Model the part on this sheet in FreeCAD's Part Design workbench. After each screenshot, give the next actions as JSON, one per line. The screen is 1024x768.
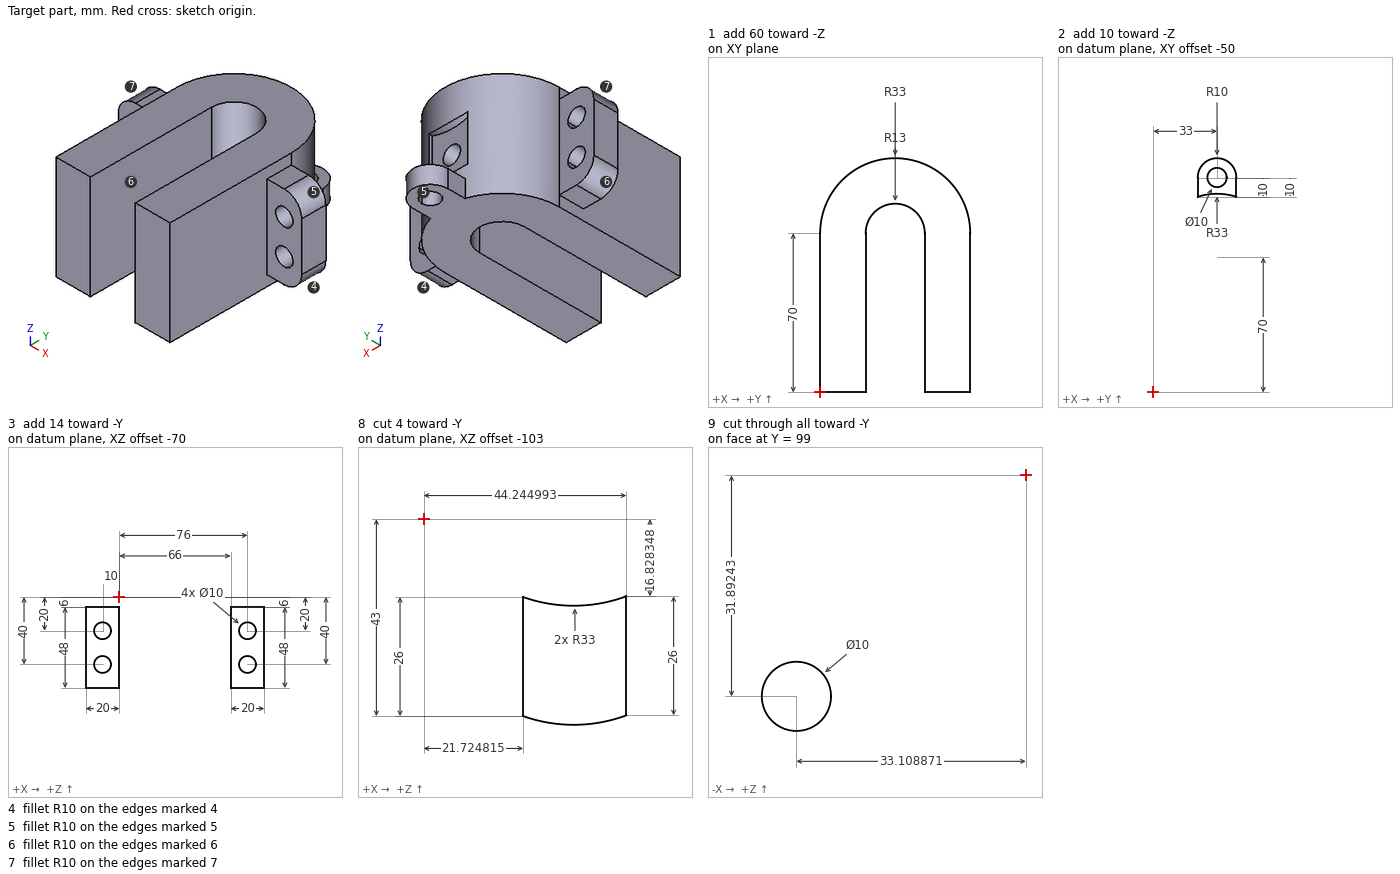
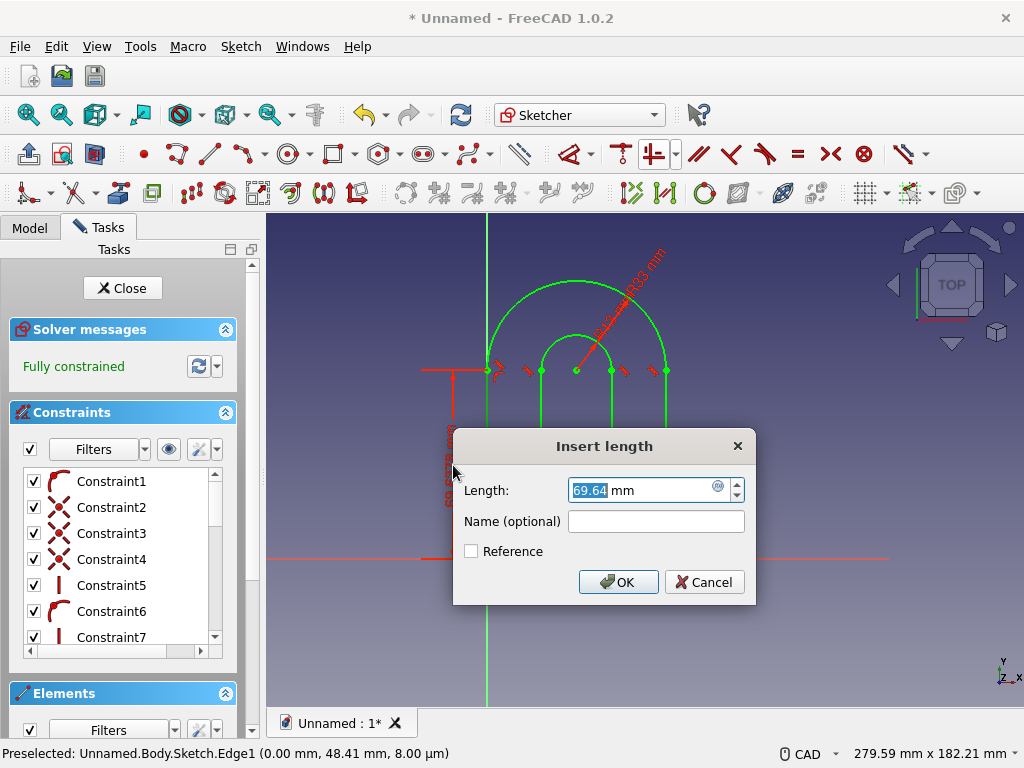
{"action": "type", "text": "70"}
{"action": "key", "text": "Return"}
{"action": "key", "text": "Escape"}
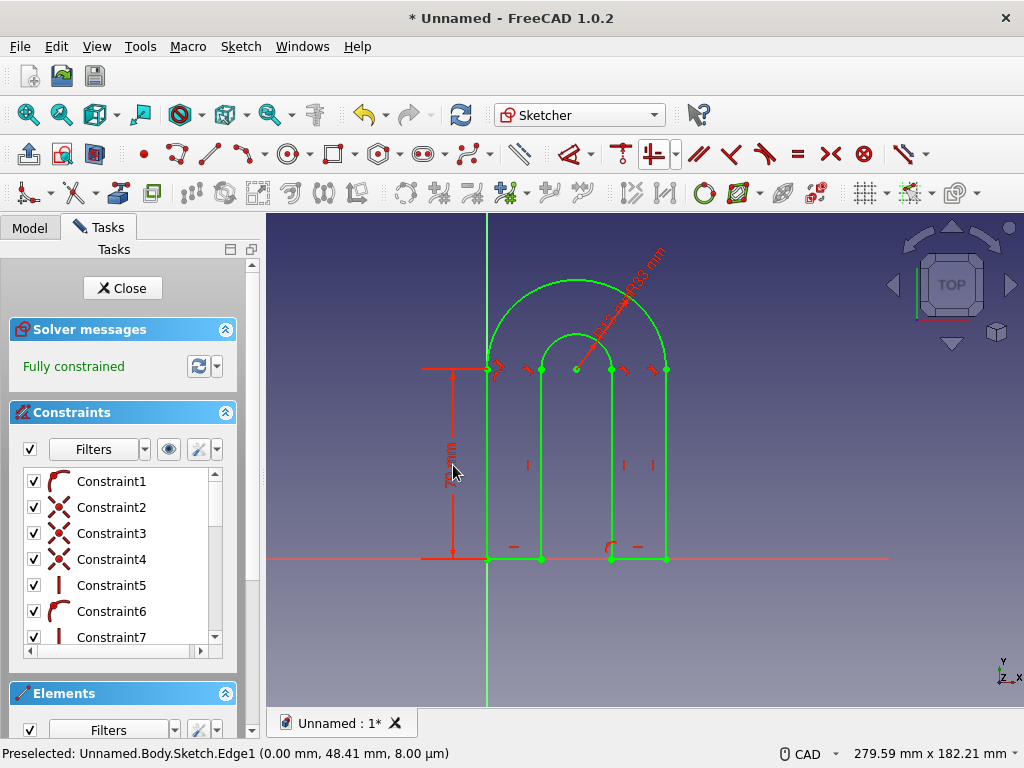
{"action": "left_click", "coordinate": [123, 288]}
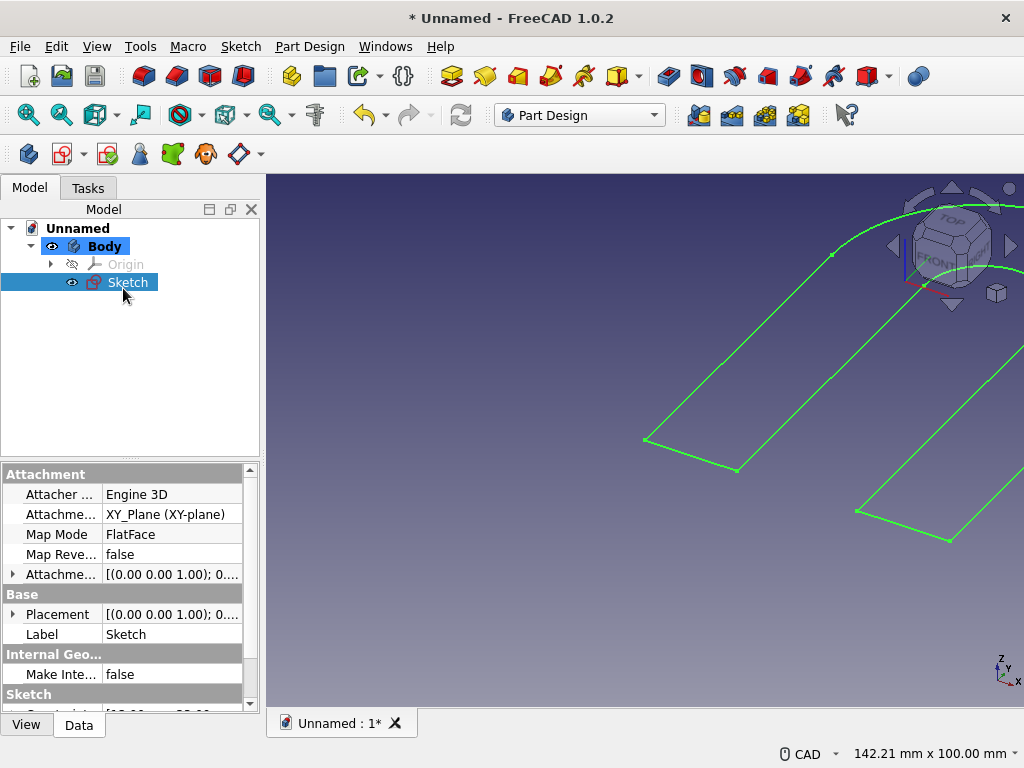
{"action": "left_click", "coordinate": [452, 76]}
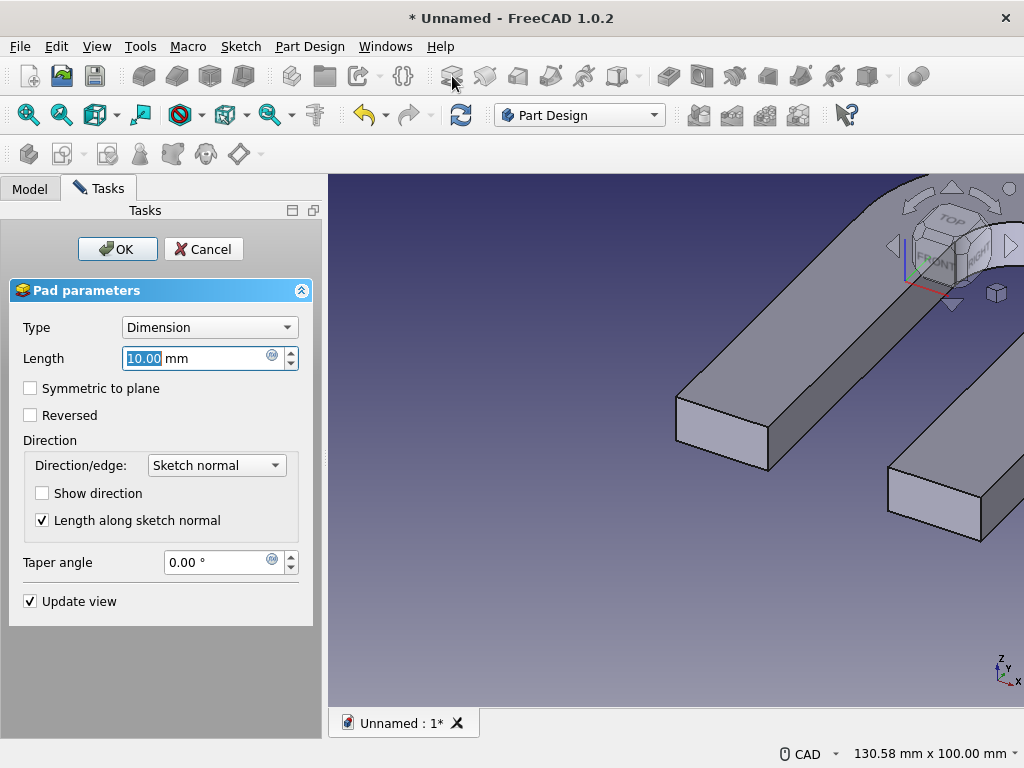
{"action": "type", "text": "60"}
{"action": "key", "text": "Tab"}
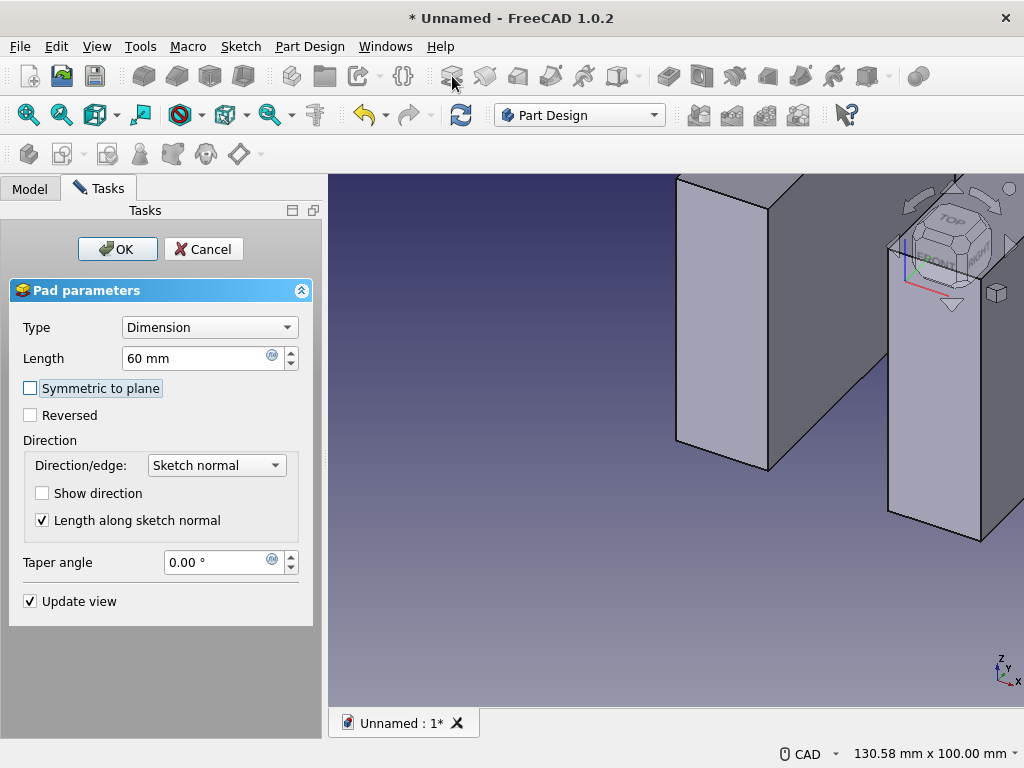
{"action": "left_click", "coordinate": [31, 415]}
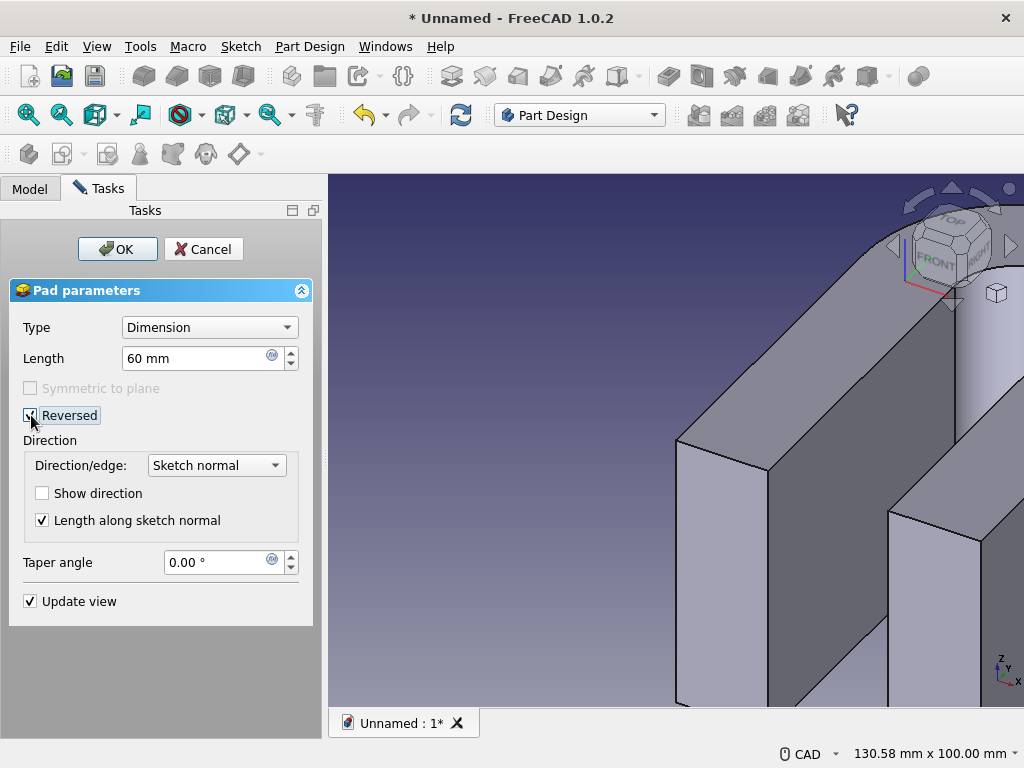
{"action": "left_click", "coordinate": [118, 249]}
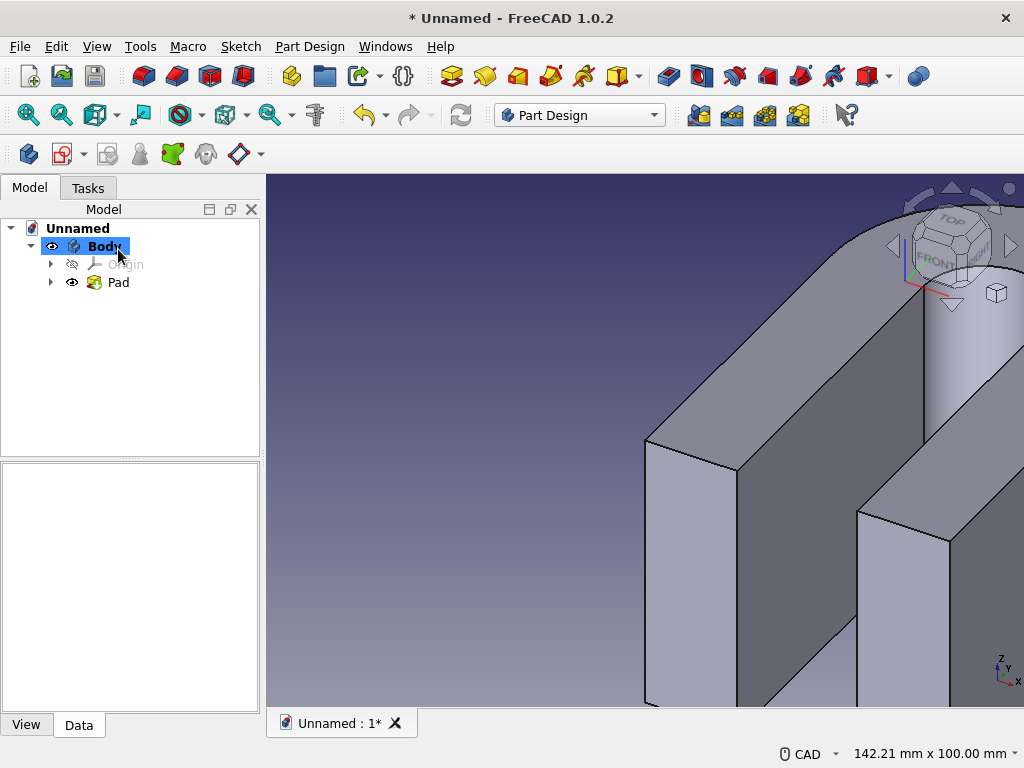
{"action": "left_click", "coordinate": [29, 116]}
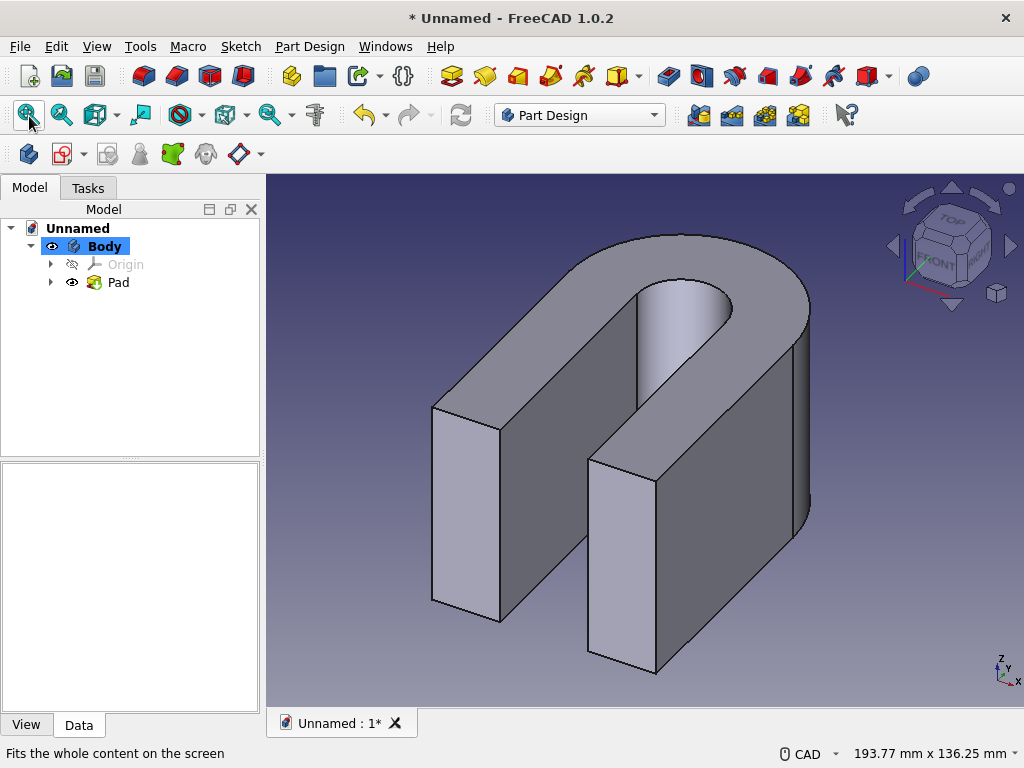
{"action": "left_click", "coordinate": [51, 264]}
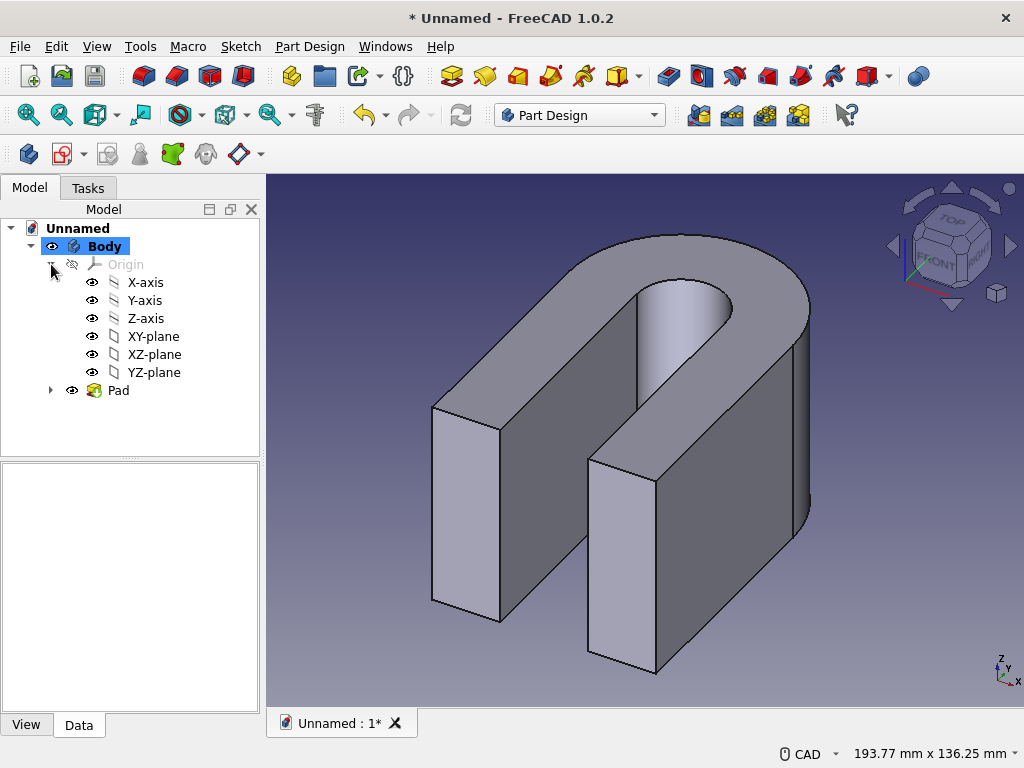
{"action": "left_click", "coordinate": [137, 336]}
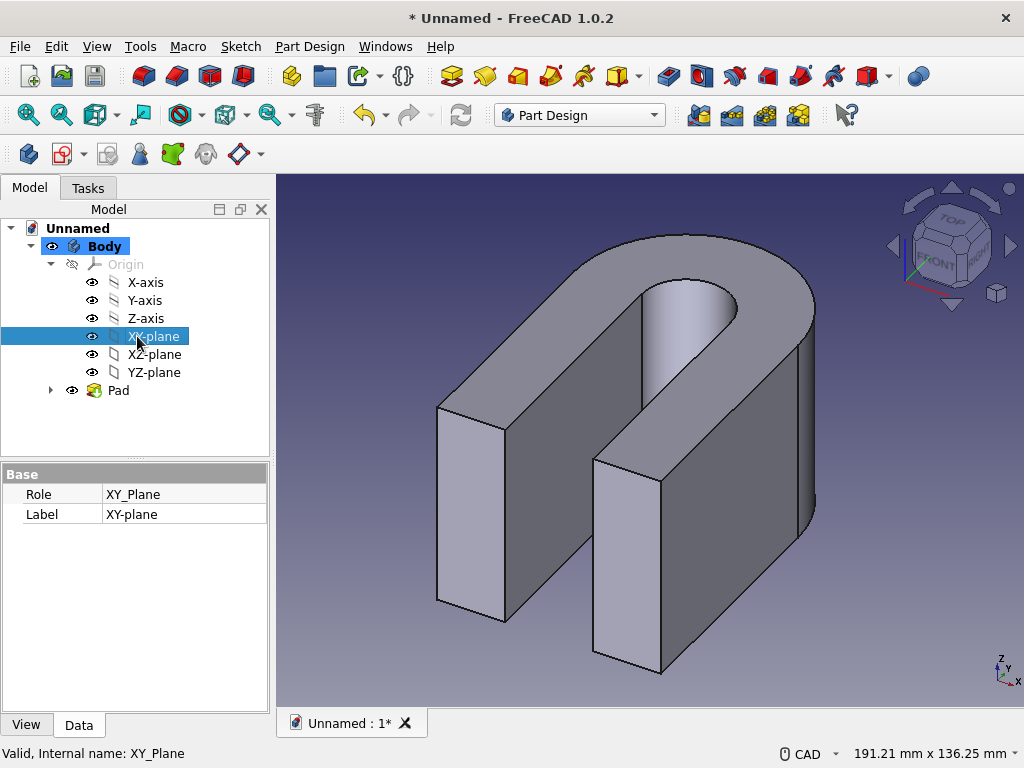
{"action": "left_click", "coordinate": [238, 154]}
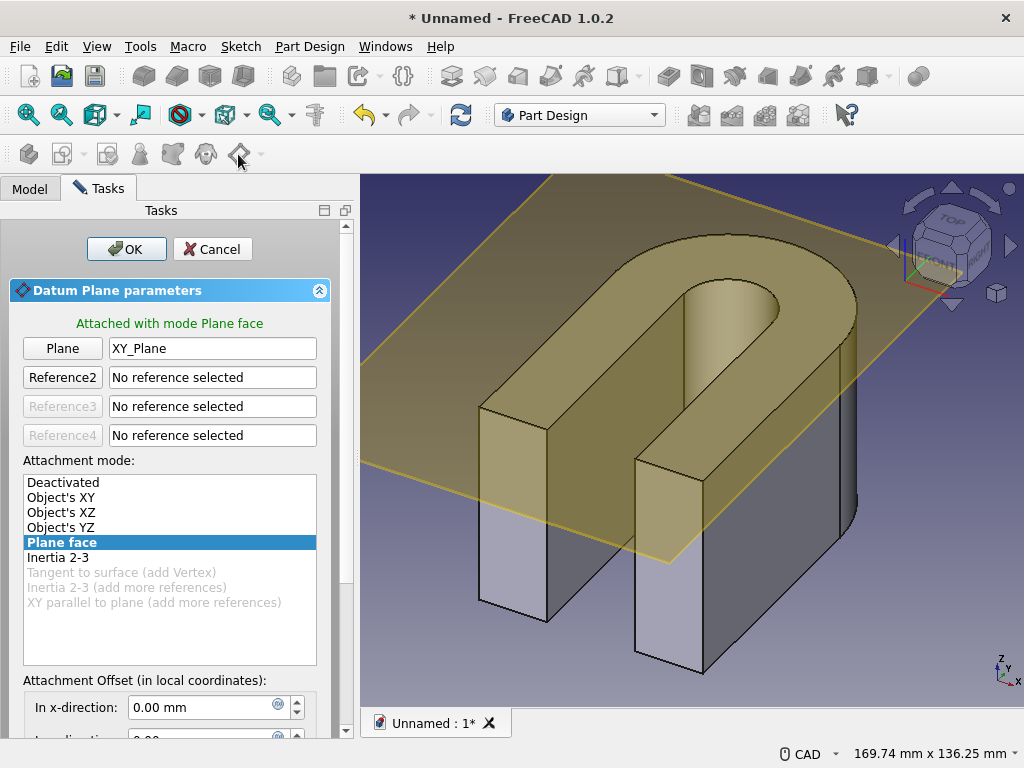
{"action": "scroll", "coordinate": [346, 479], "scroll_direction": "down", "scroll_amount": 2}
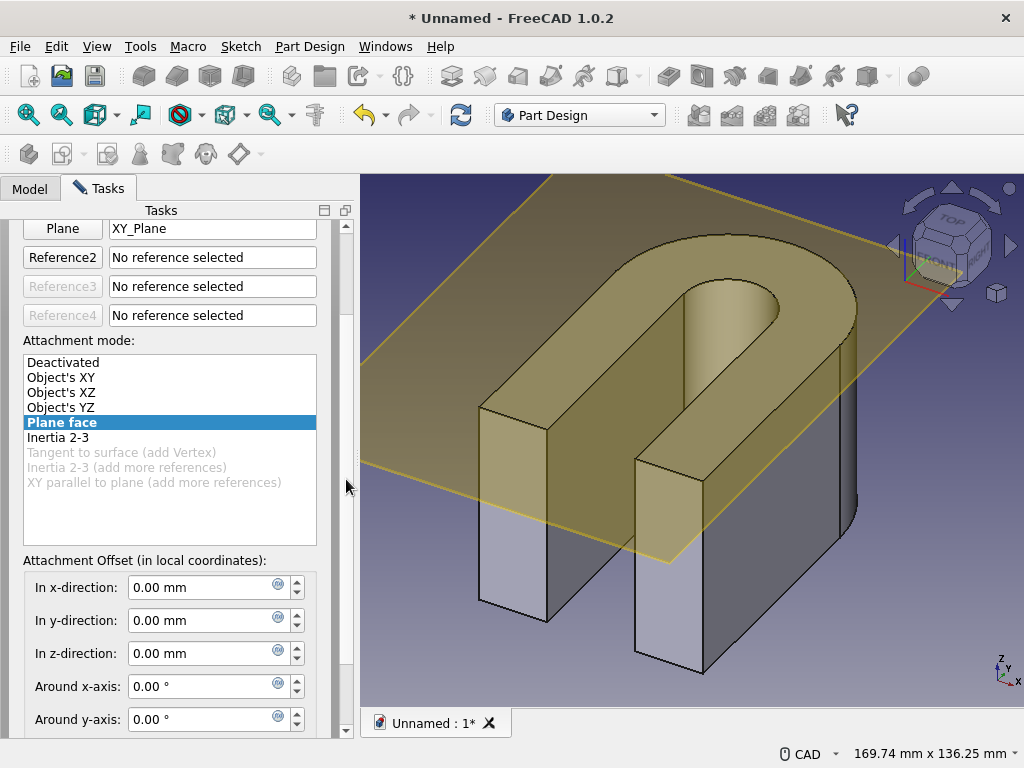
{"action": "triple_click", "coordinate": [210, 654]}